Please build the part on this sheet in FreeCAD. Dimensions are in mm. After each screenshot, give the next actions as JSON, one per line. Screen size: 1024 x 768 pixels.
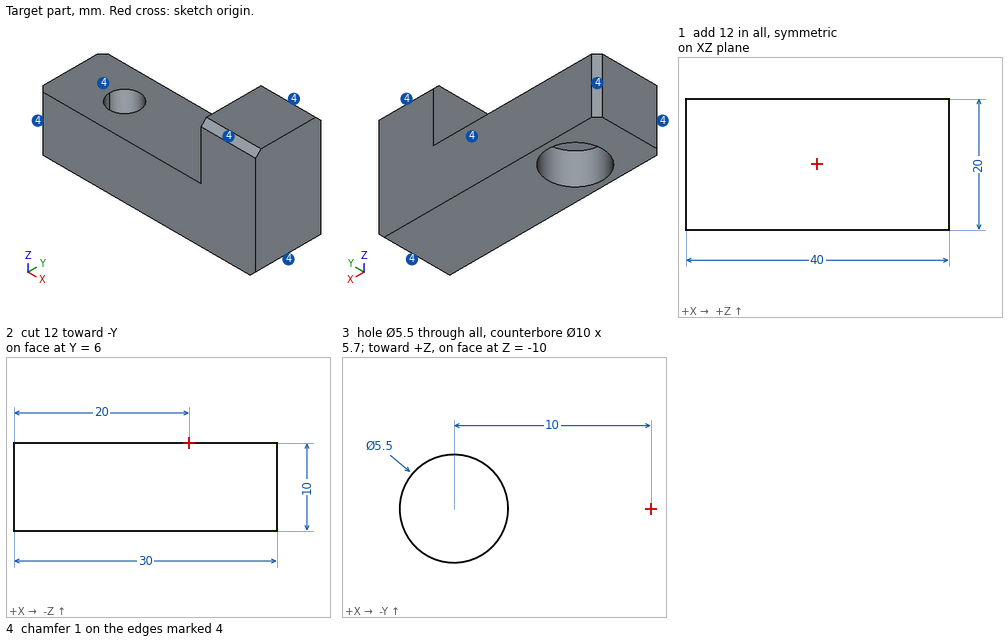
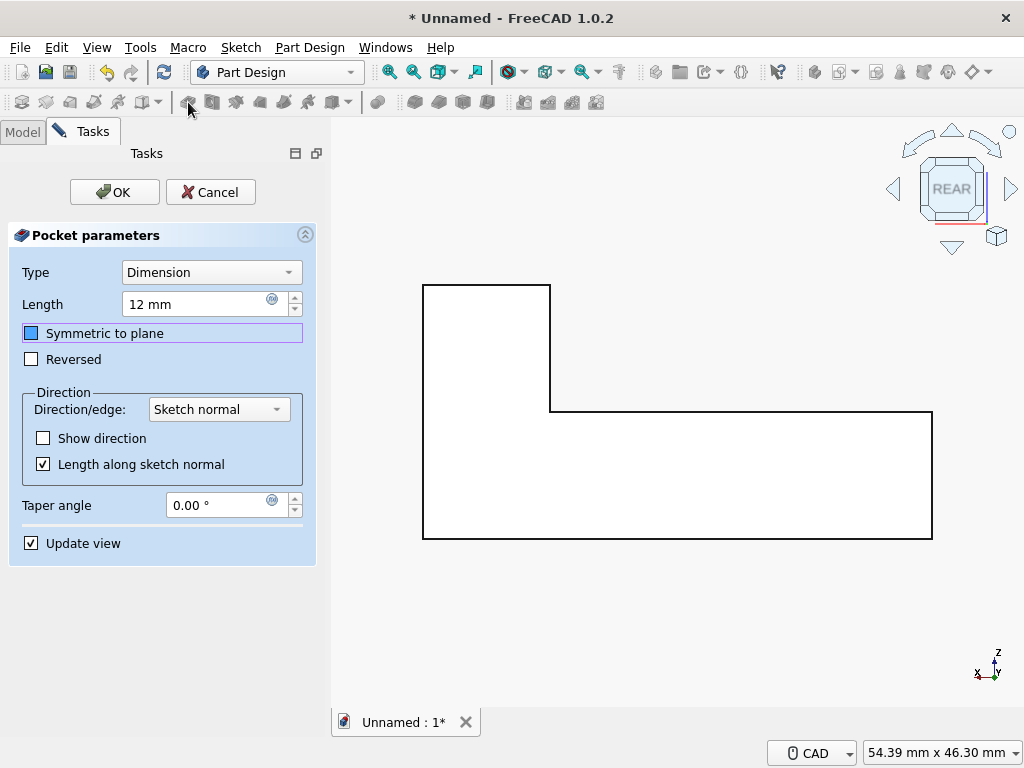
{"action": "left_click", "coordinate": [115, 192]}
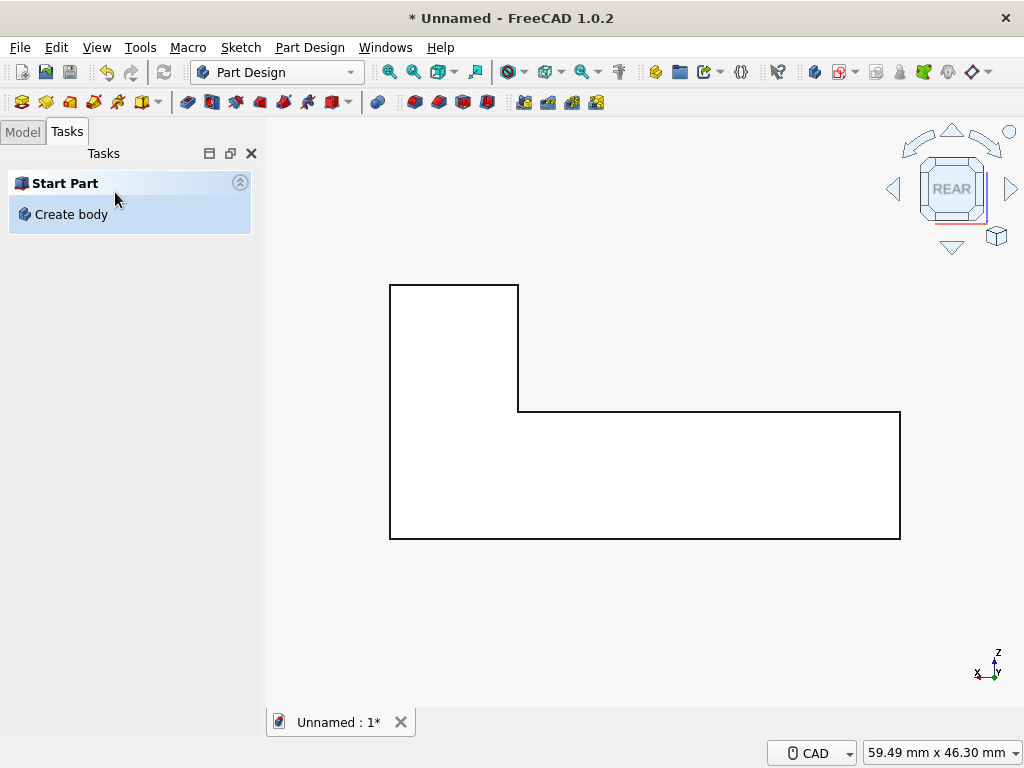
{"action": "key", "text": "5"}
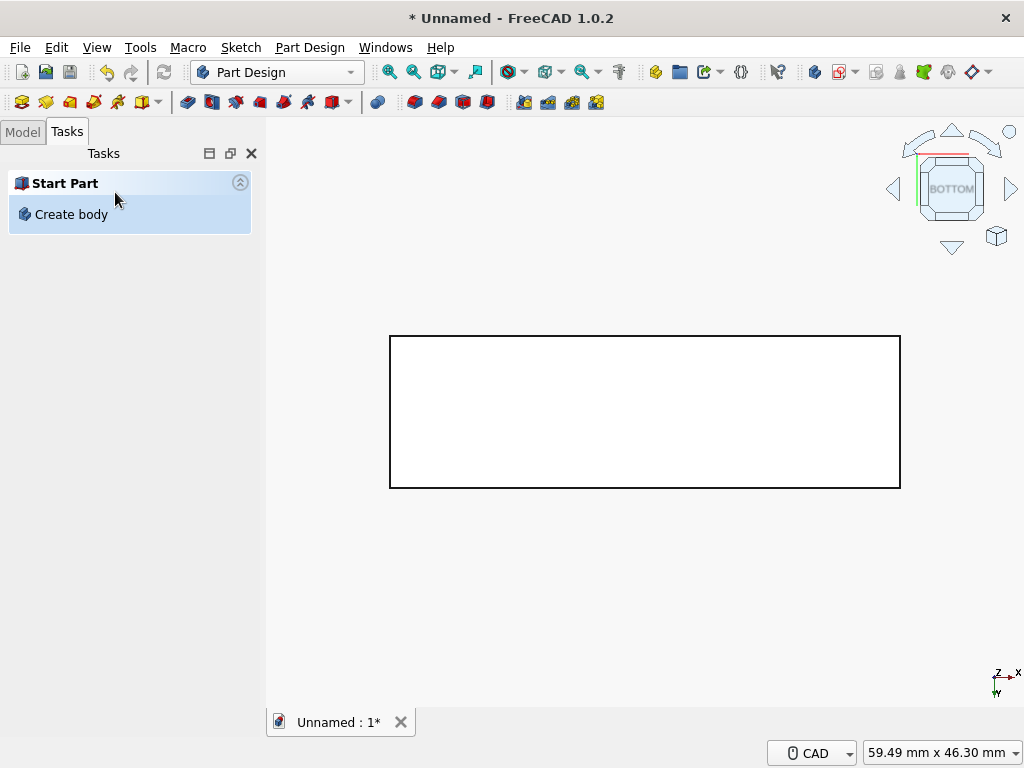
{"action": "left_click", "coordinate": [791, 411]}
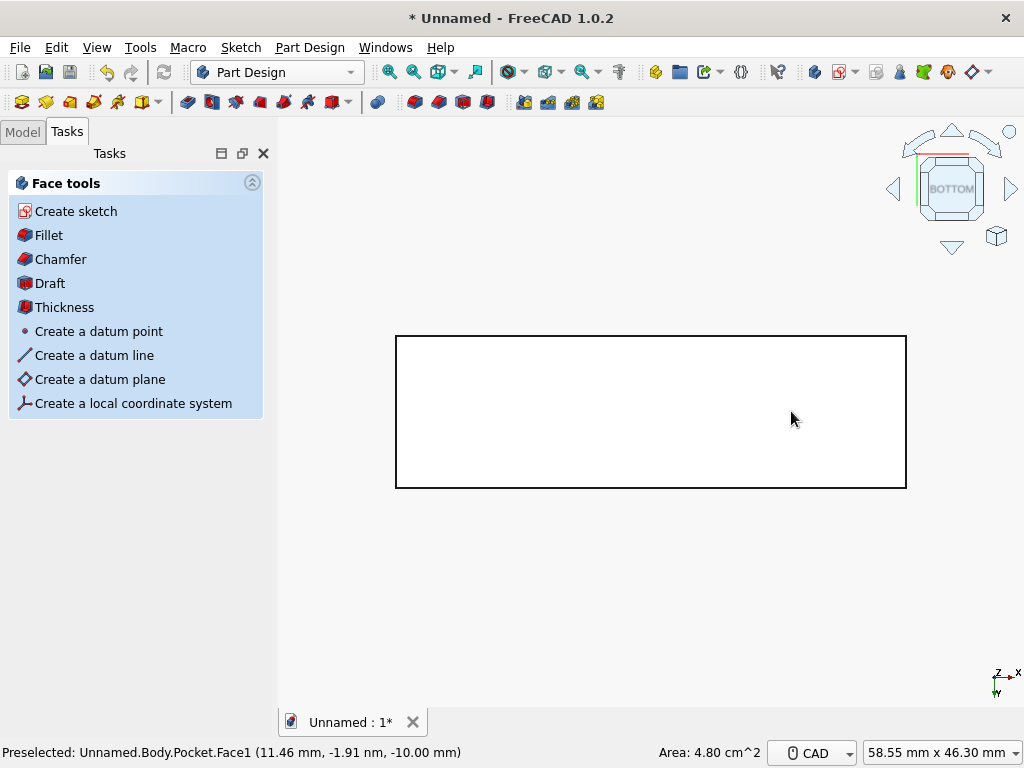
{"action": "left_click", "coordinate": [840, 72]}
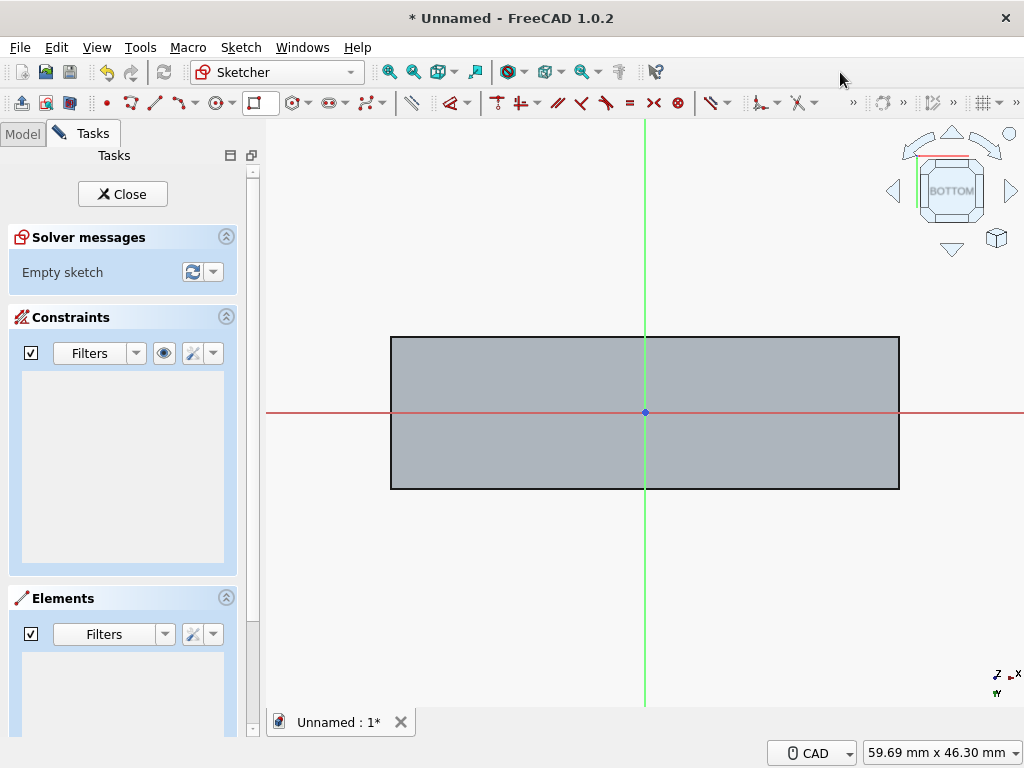
{"action": "scroll", "coordinate": [557, 413], "scroll_direction": "up", "scroll_amount": 5}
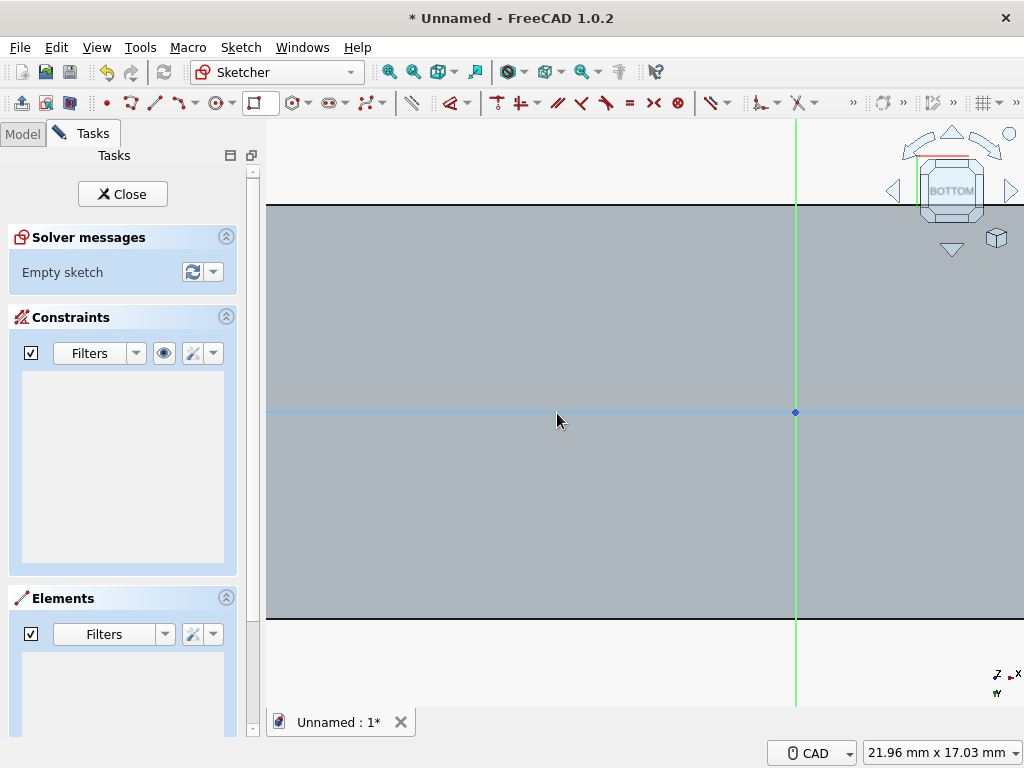
{"action": "key", "text": "g c"}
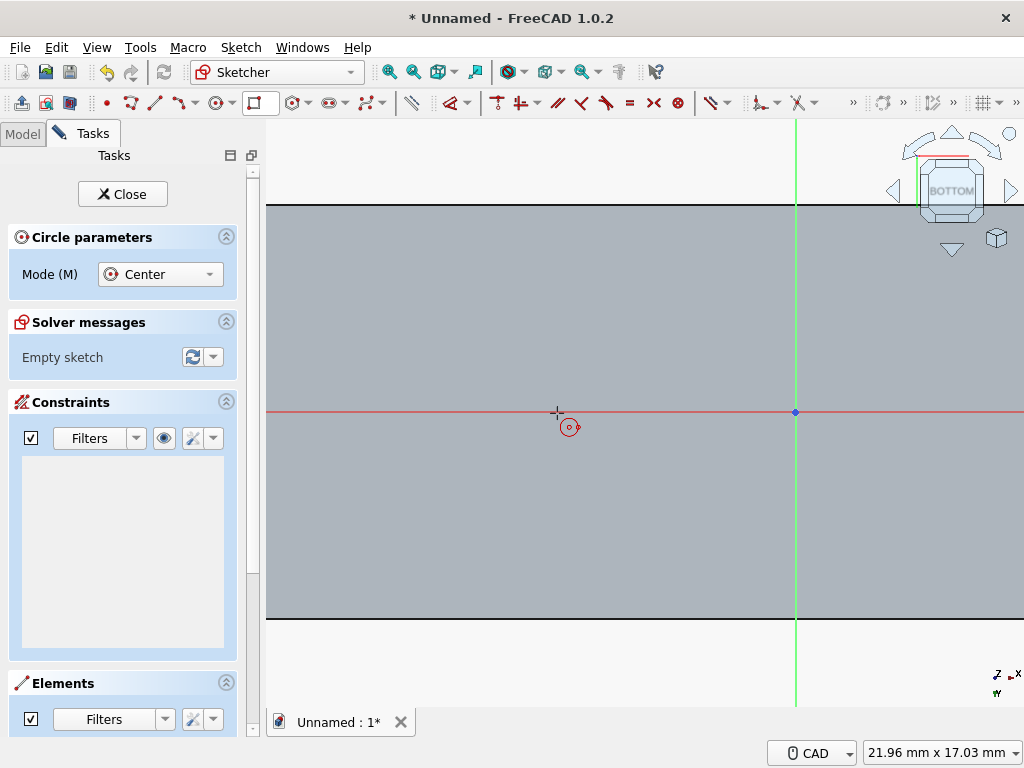
{"action": "left_click", "coordinate": [450, 412]}
{"action": "mouse_move", "coordinate": [517, 345]}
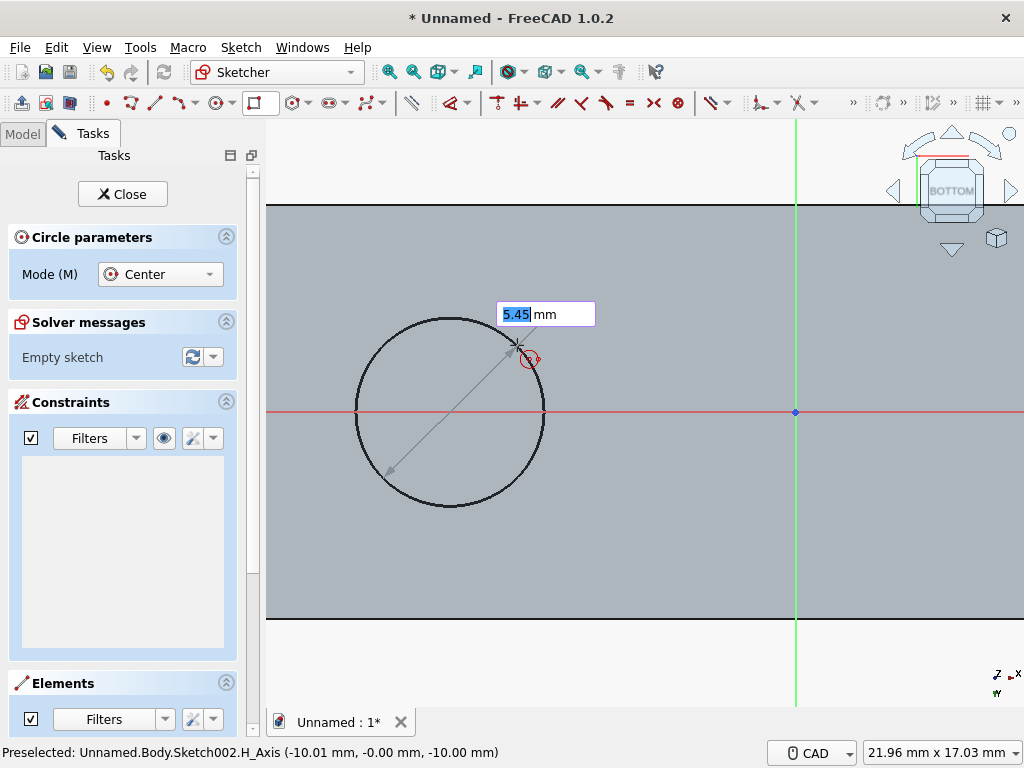
{"action": "type", "text": "5.5"}
{"action": "key", "text": "Return"}
{"action": "key", "text": "Escape"}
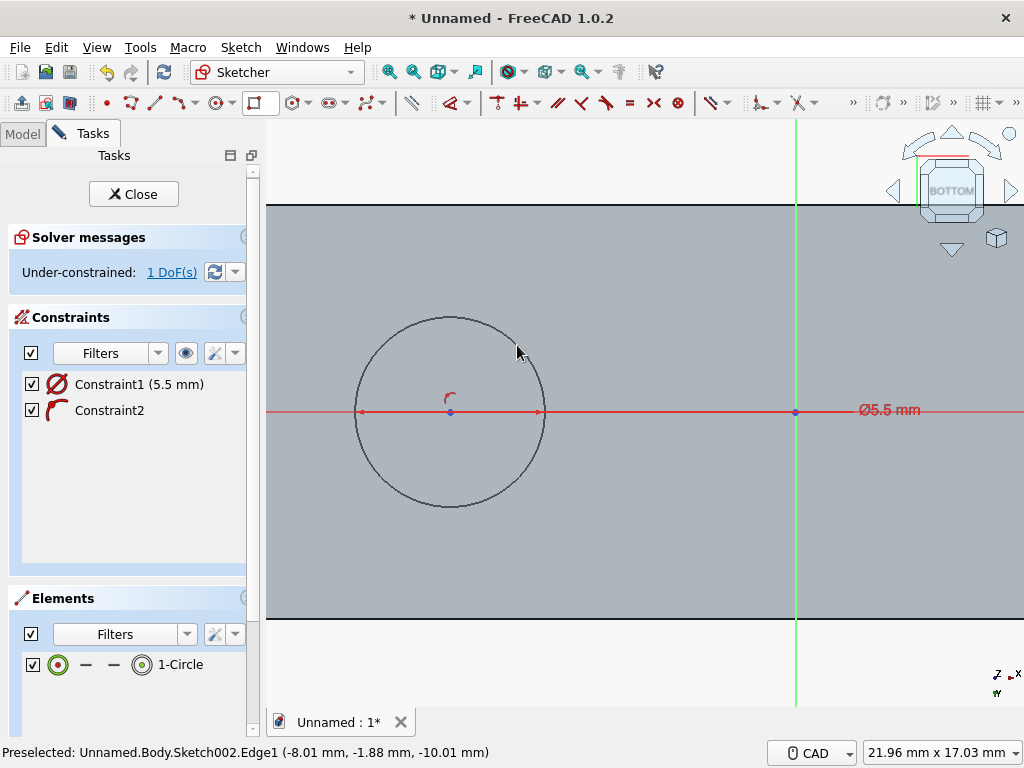
{"action": "left_click", "coordinate": [450, 412]}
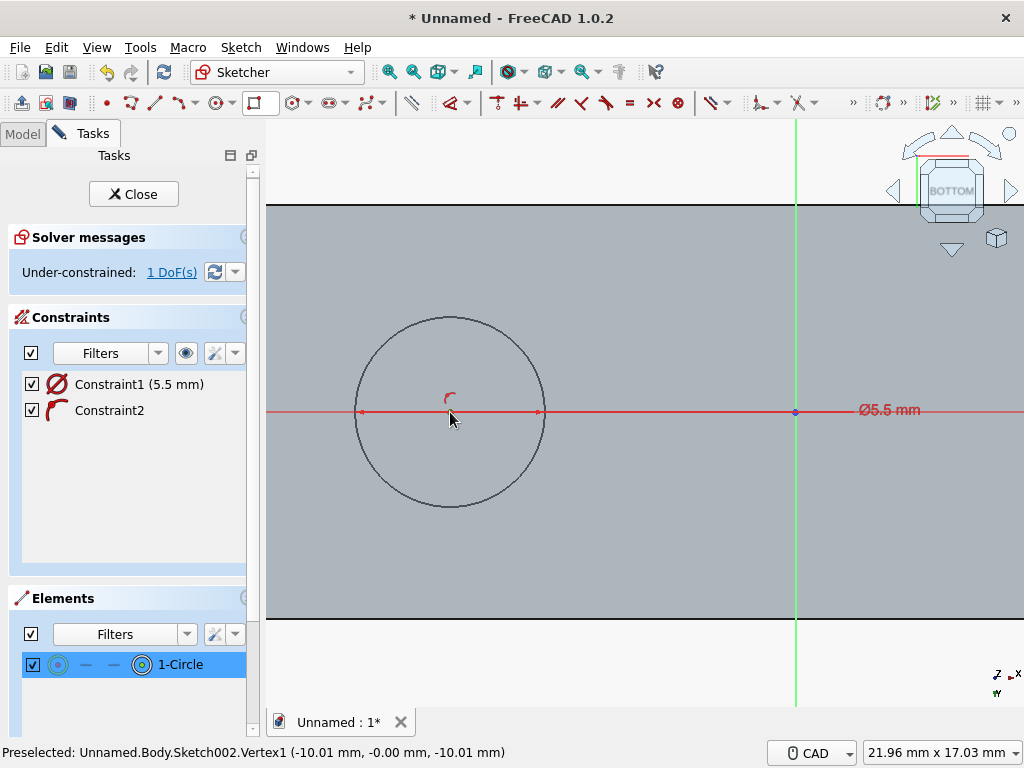
{"action": "key", "text": "l"}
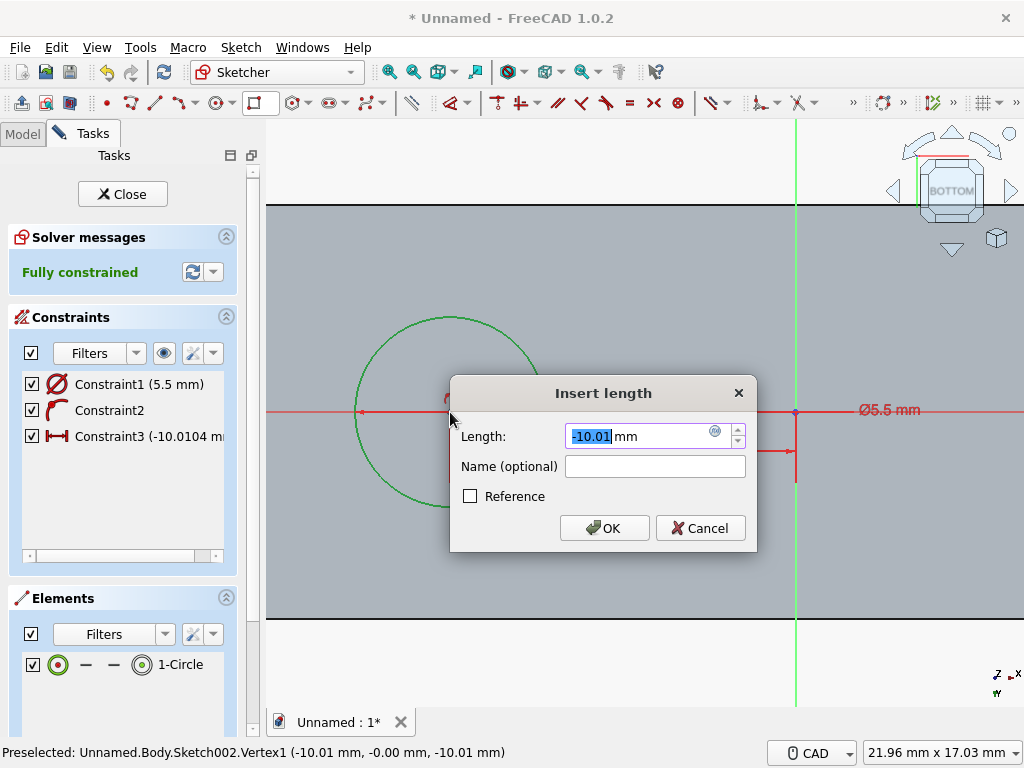
{"action": "type", "text": "-10"}
{"action": "key", "text": "Return"}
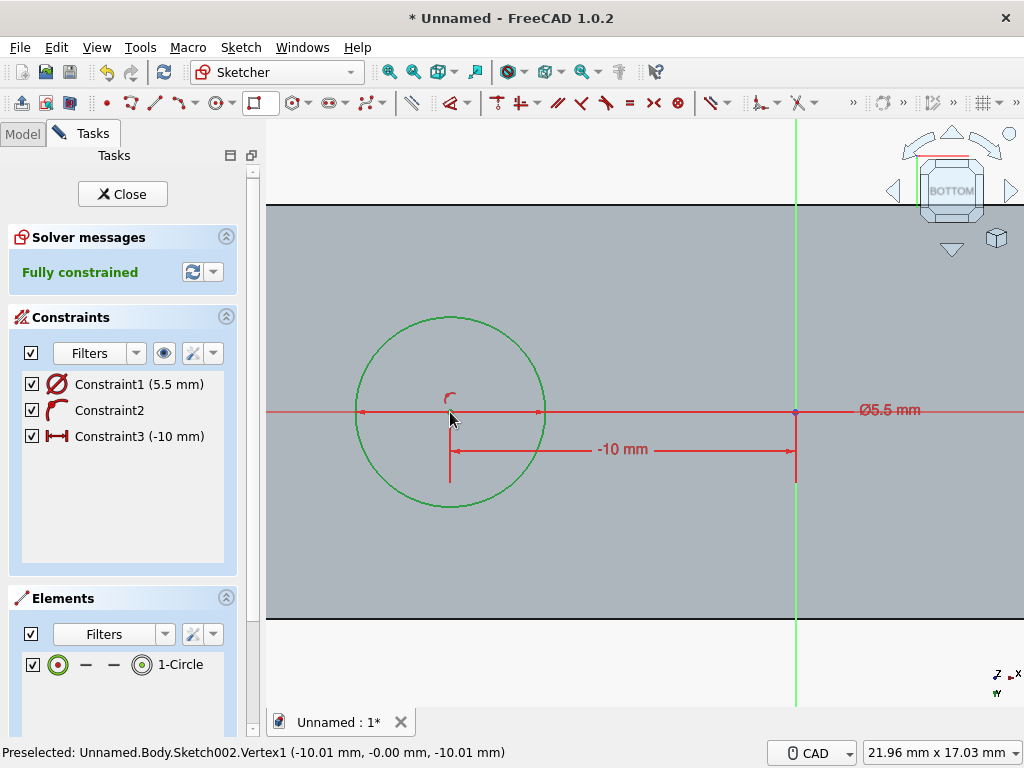
{"action": "left_click", "coordinate": [123, 194]}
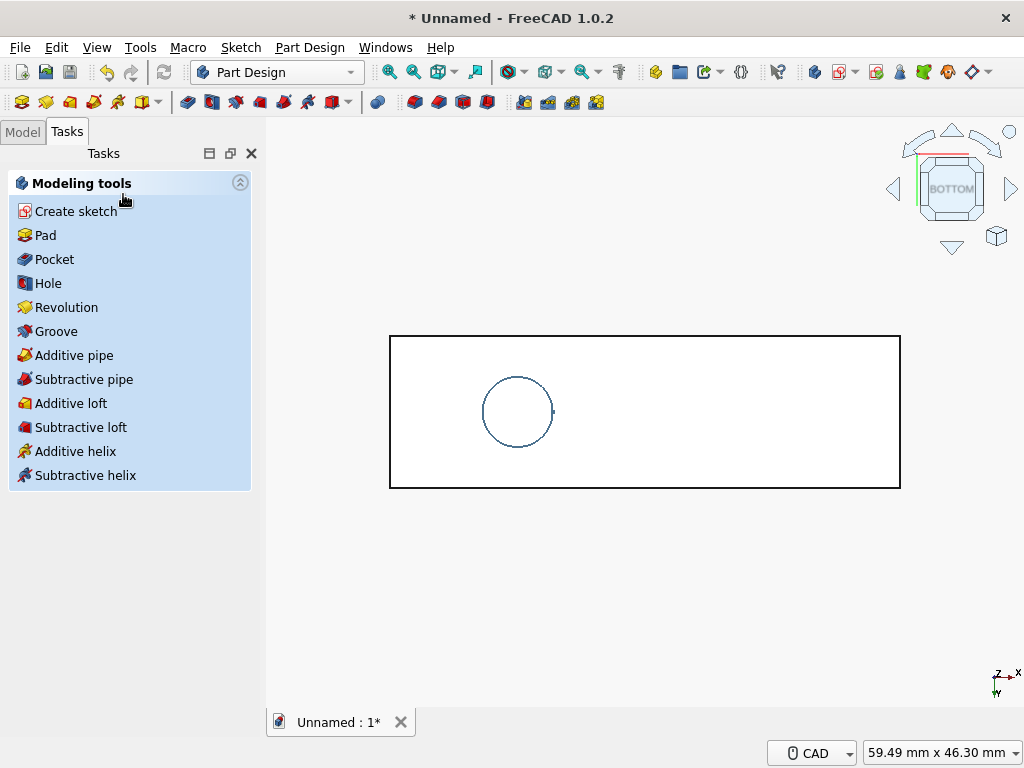
{"action": "left_click", "coordinate": [212, 102]}